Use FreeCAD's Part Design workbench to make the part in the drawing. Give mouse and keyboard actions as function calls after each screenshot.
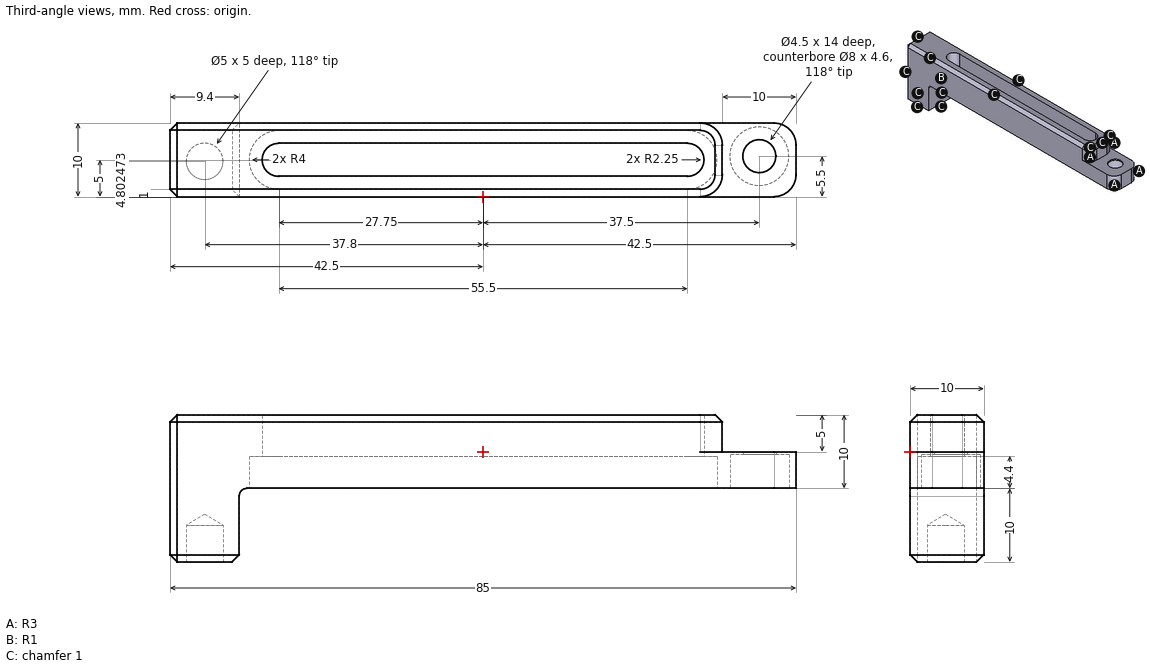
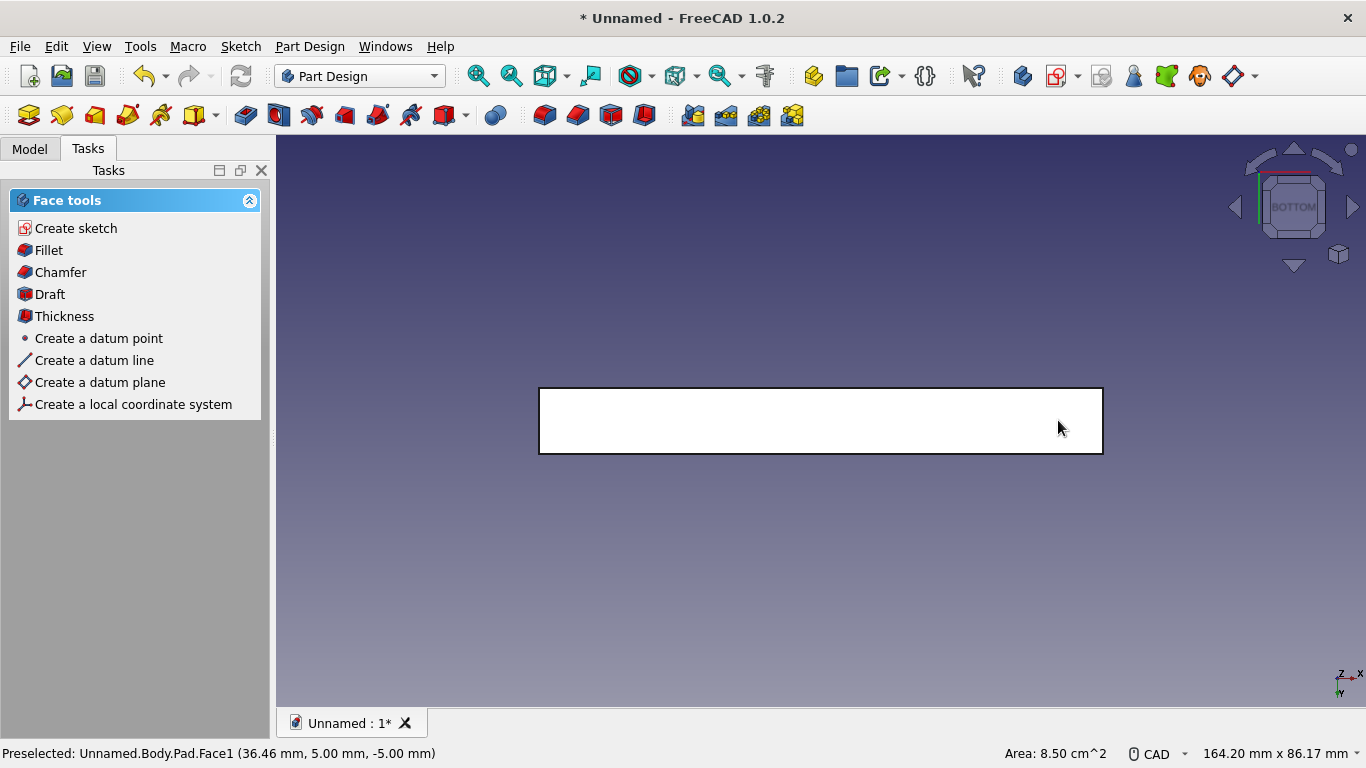
click(1056, 76)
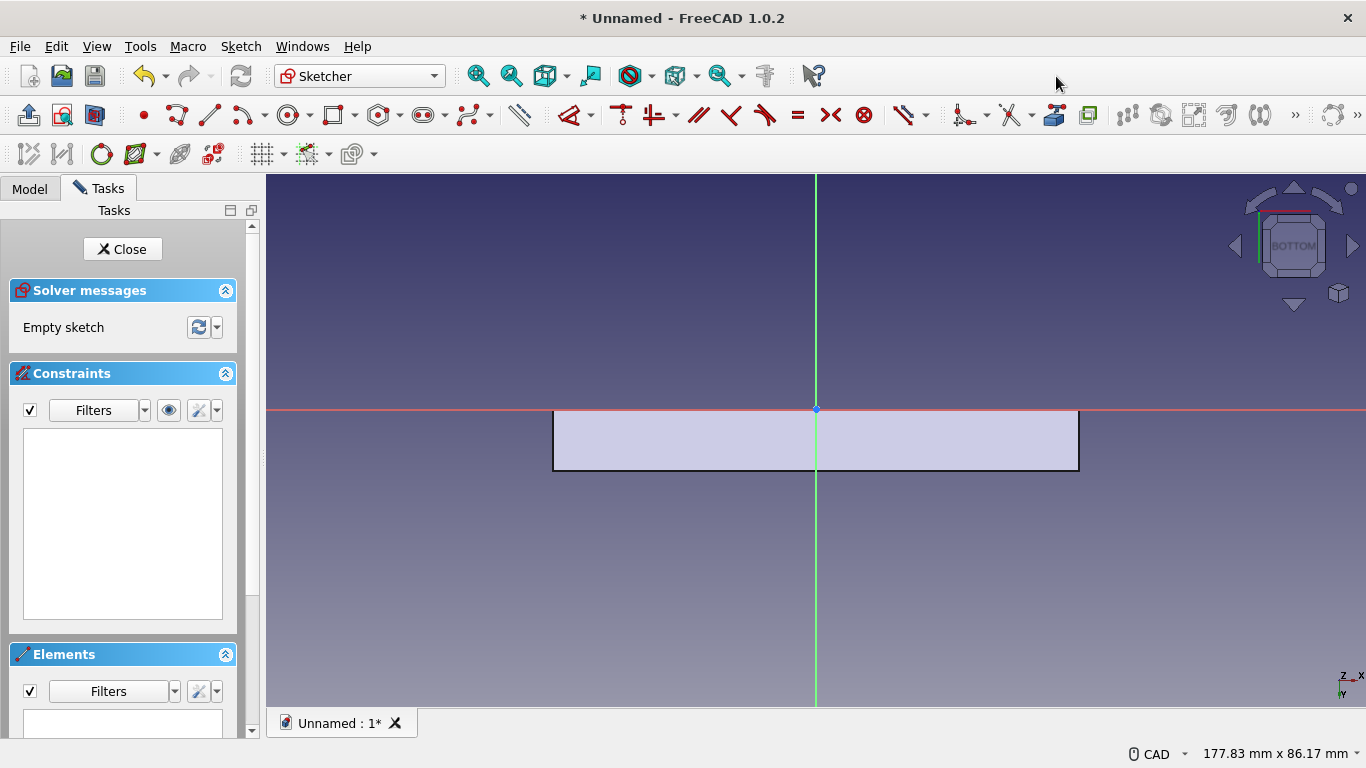
scroll(955, 431, up, 2)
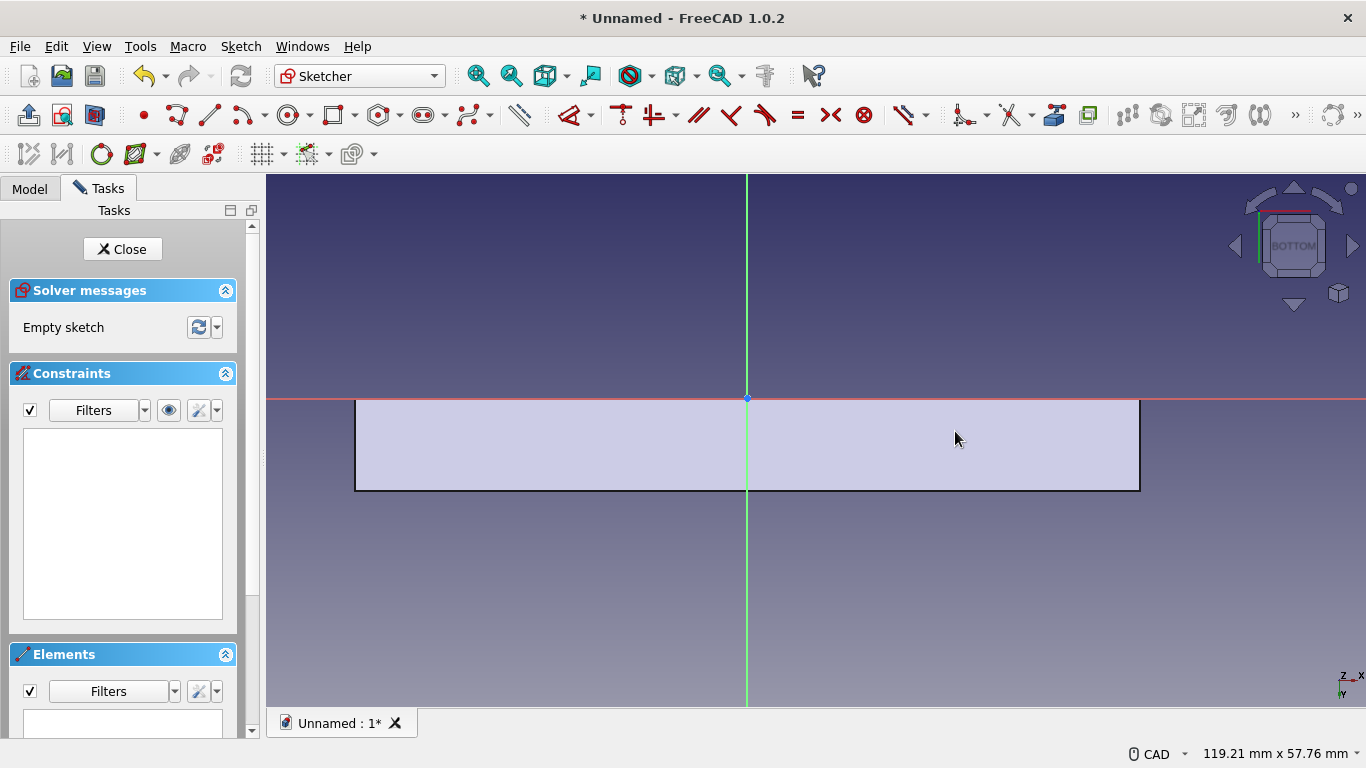
key(g)
key(s)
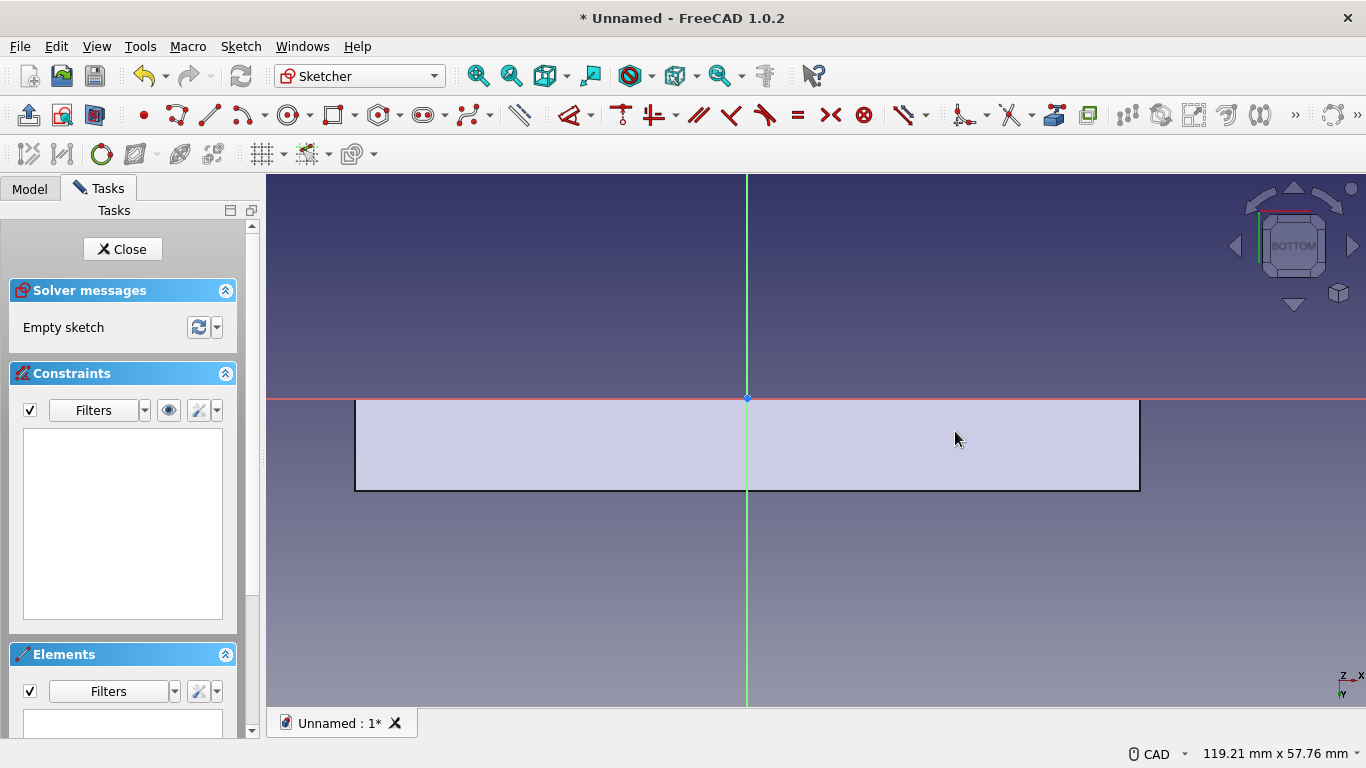
click(491, 445)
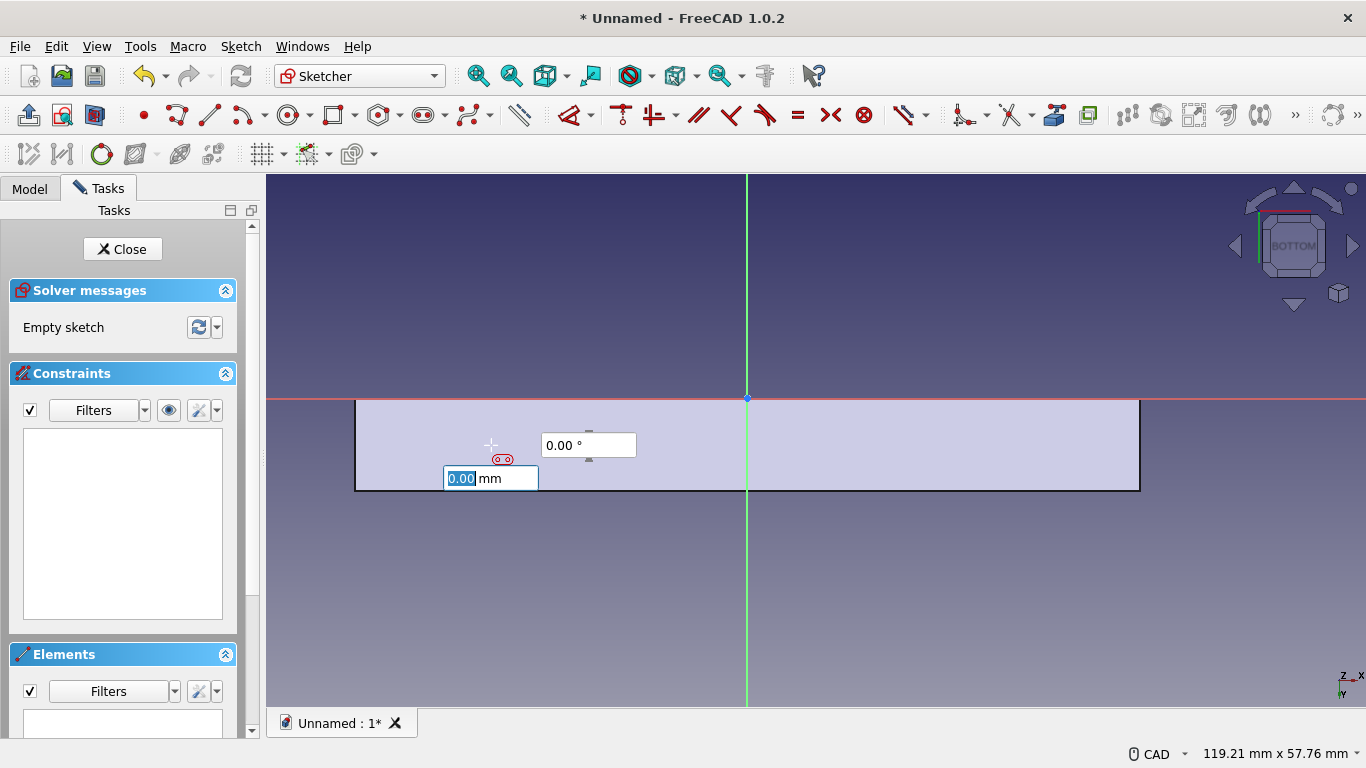
click(1003, 445)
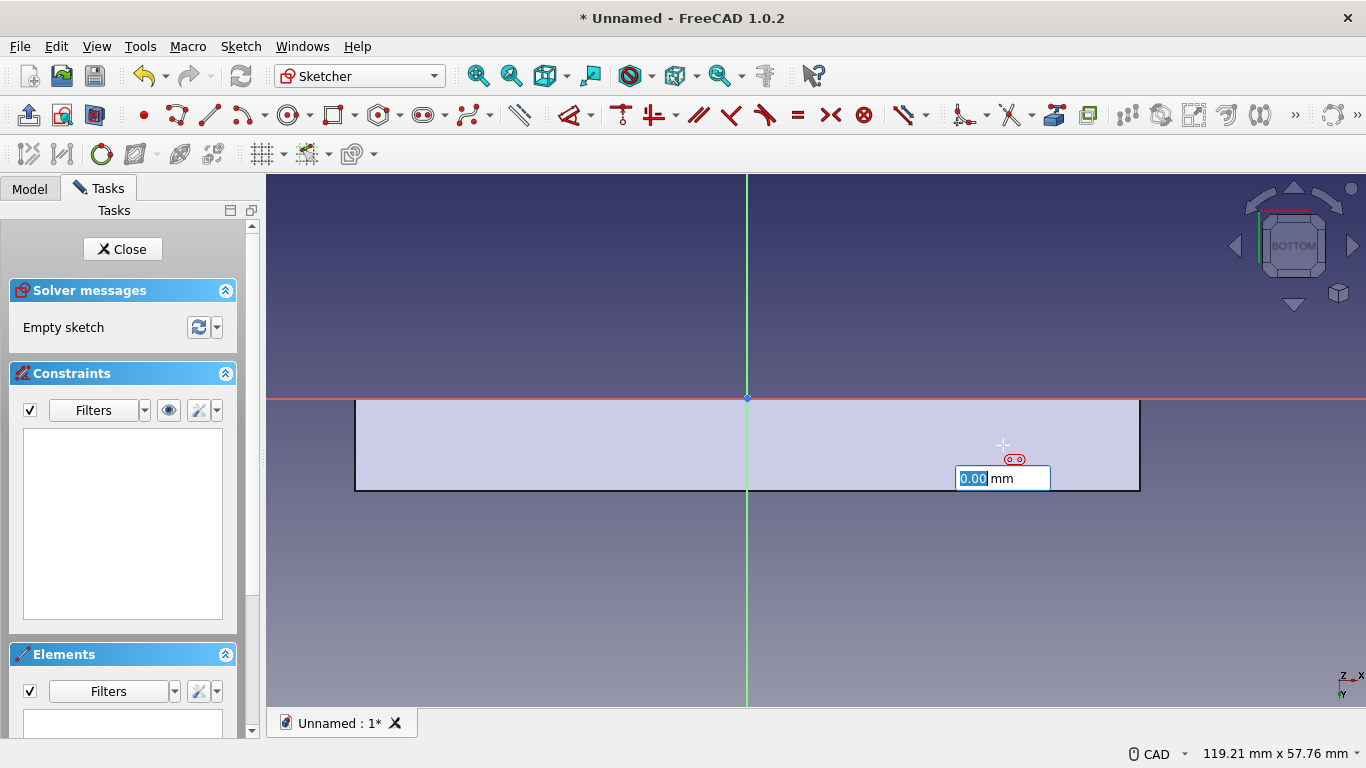
click(824, 482)
key(Escape)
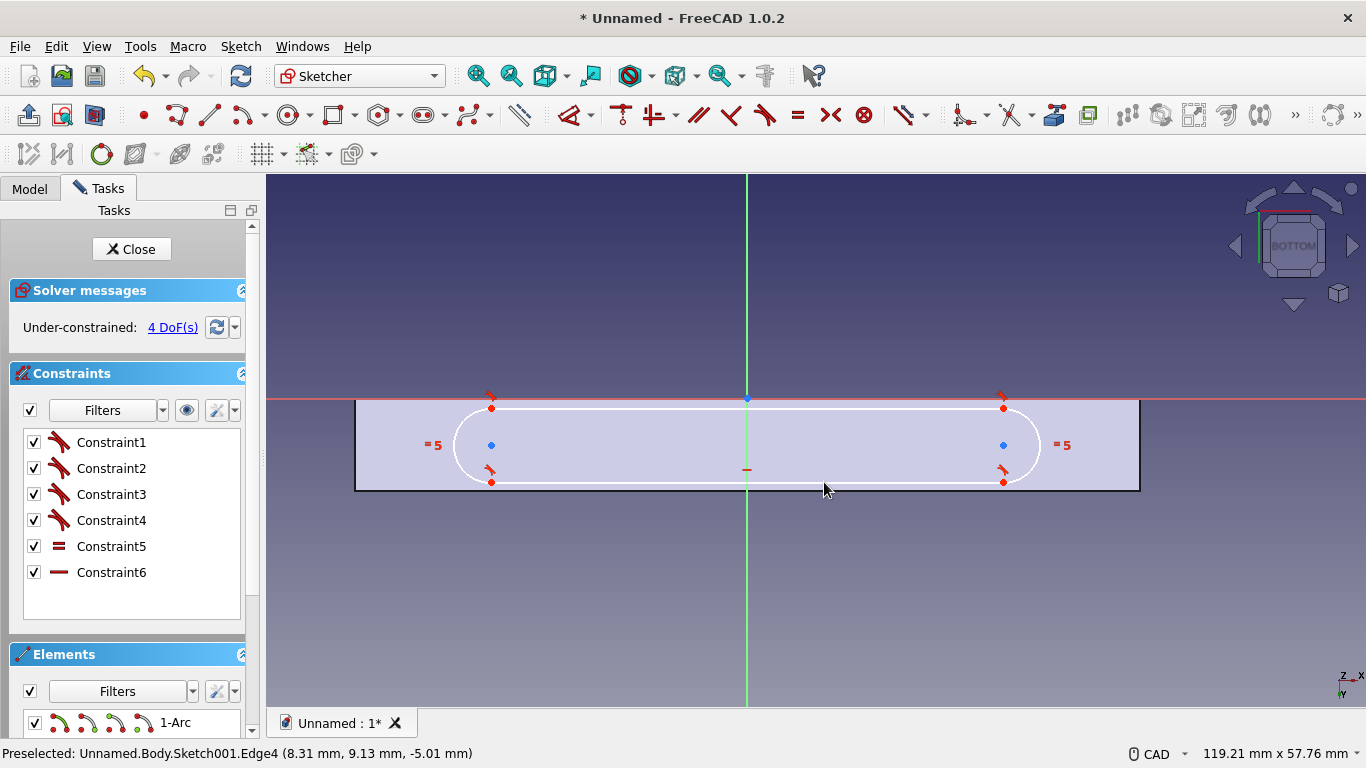
key(d)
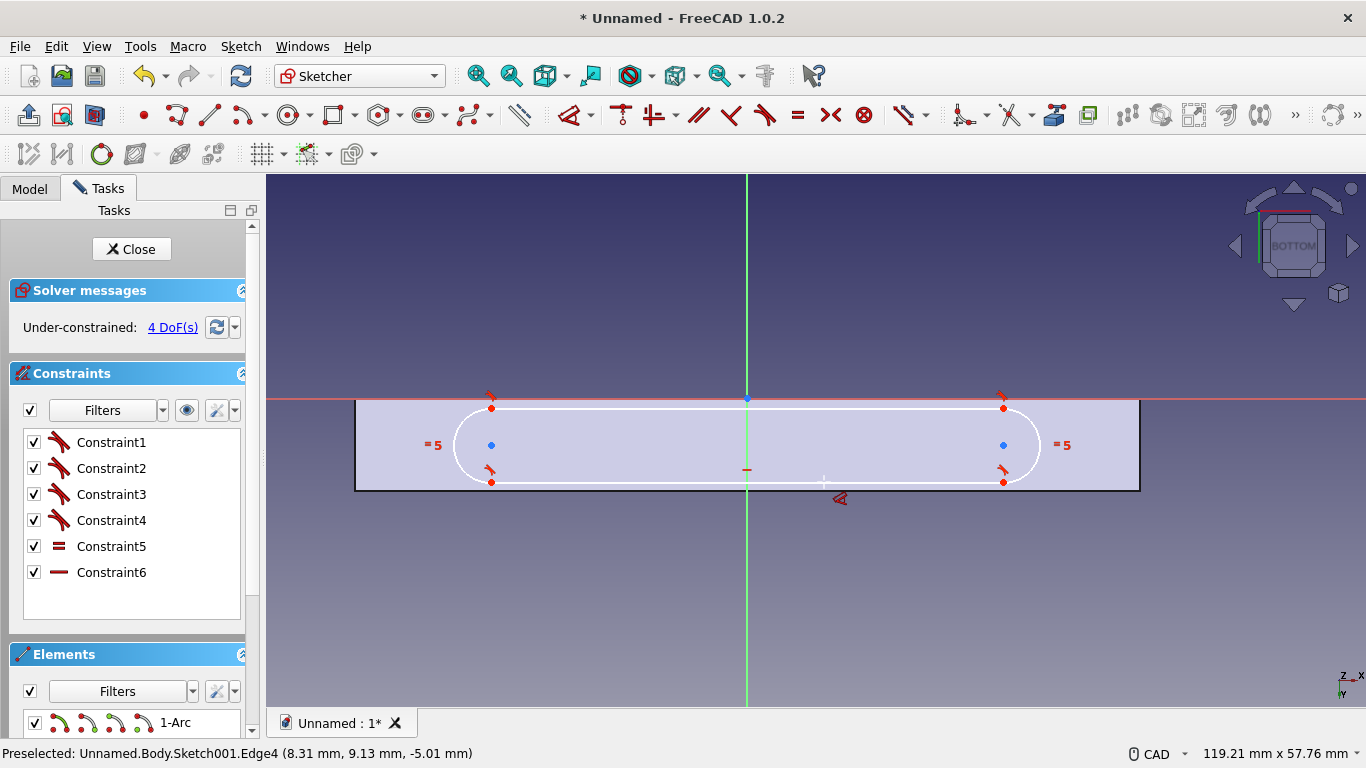
click(461, 424)
click(462, 383)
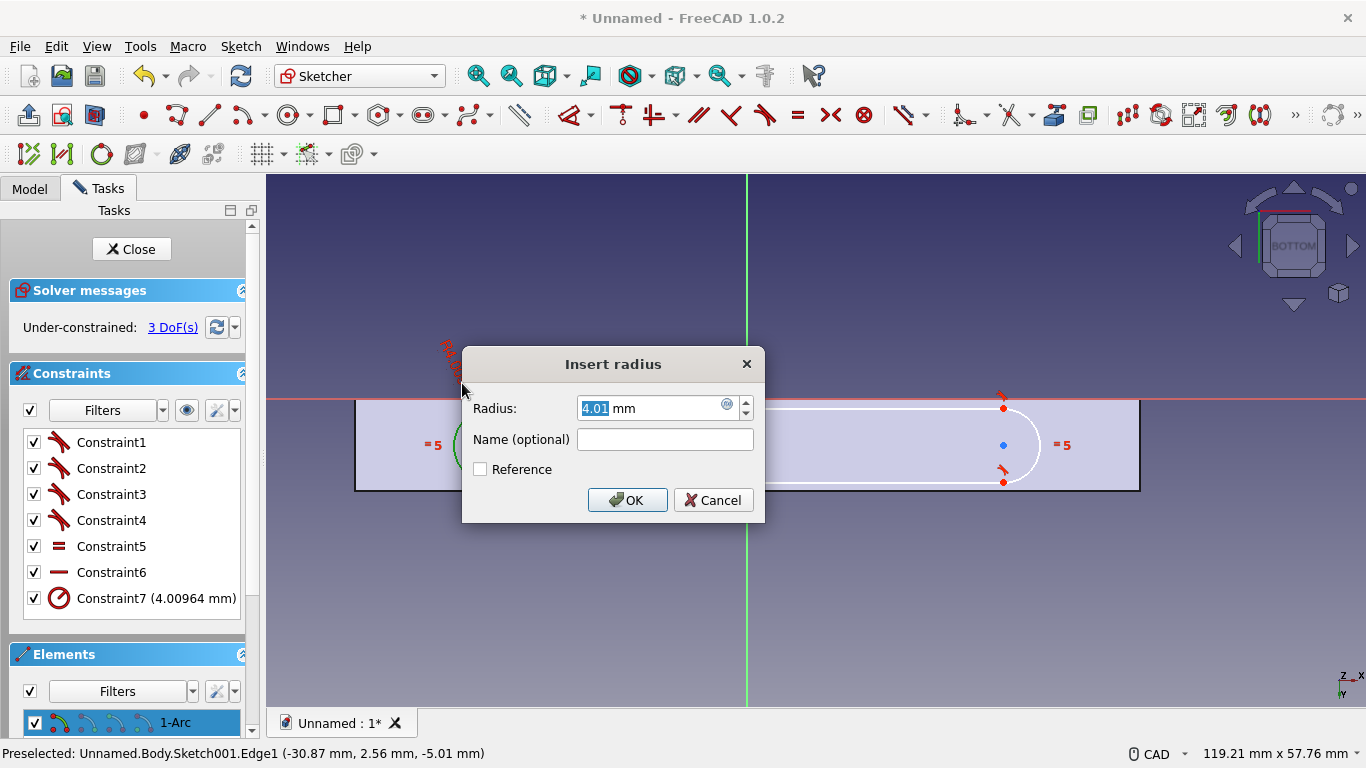
text(4)
key(Return)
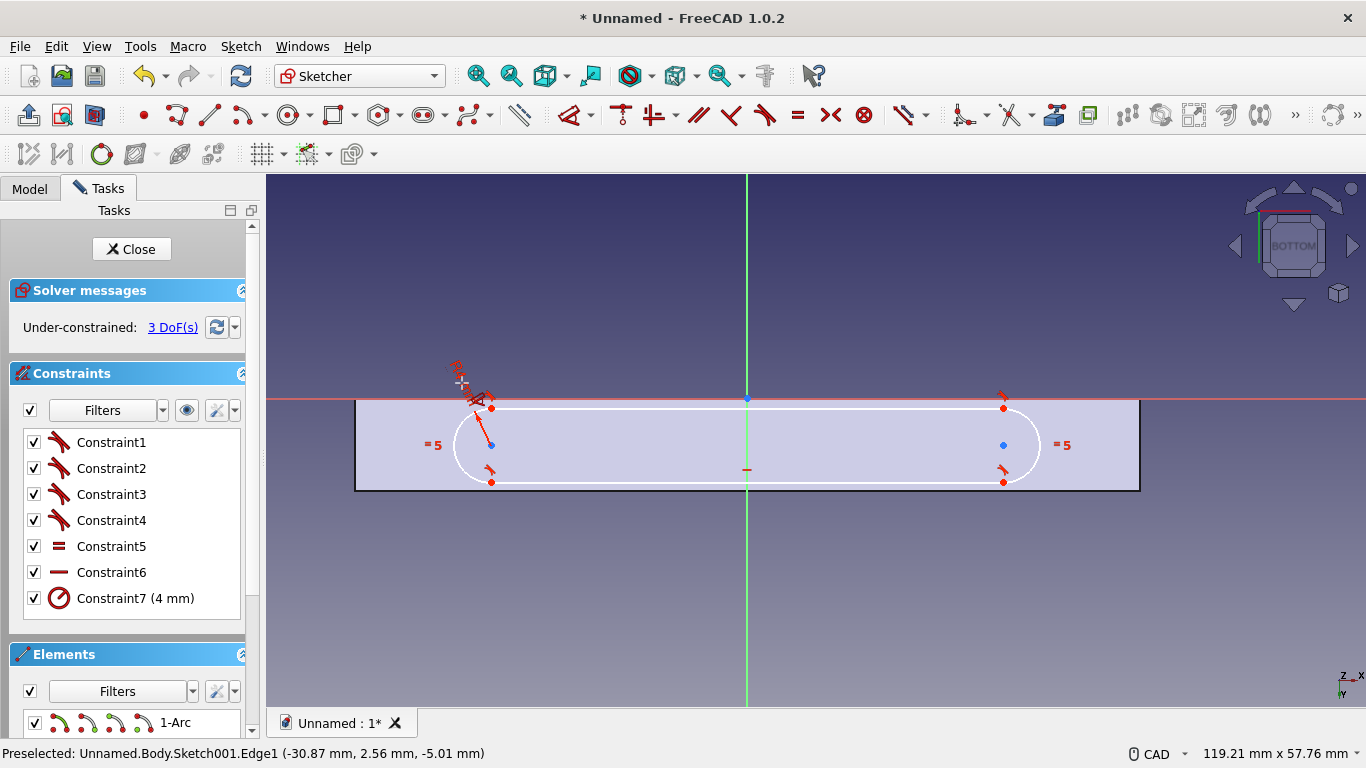
scroll(491, 409, up, 8)